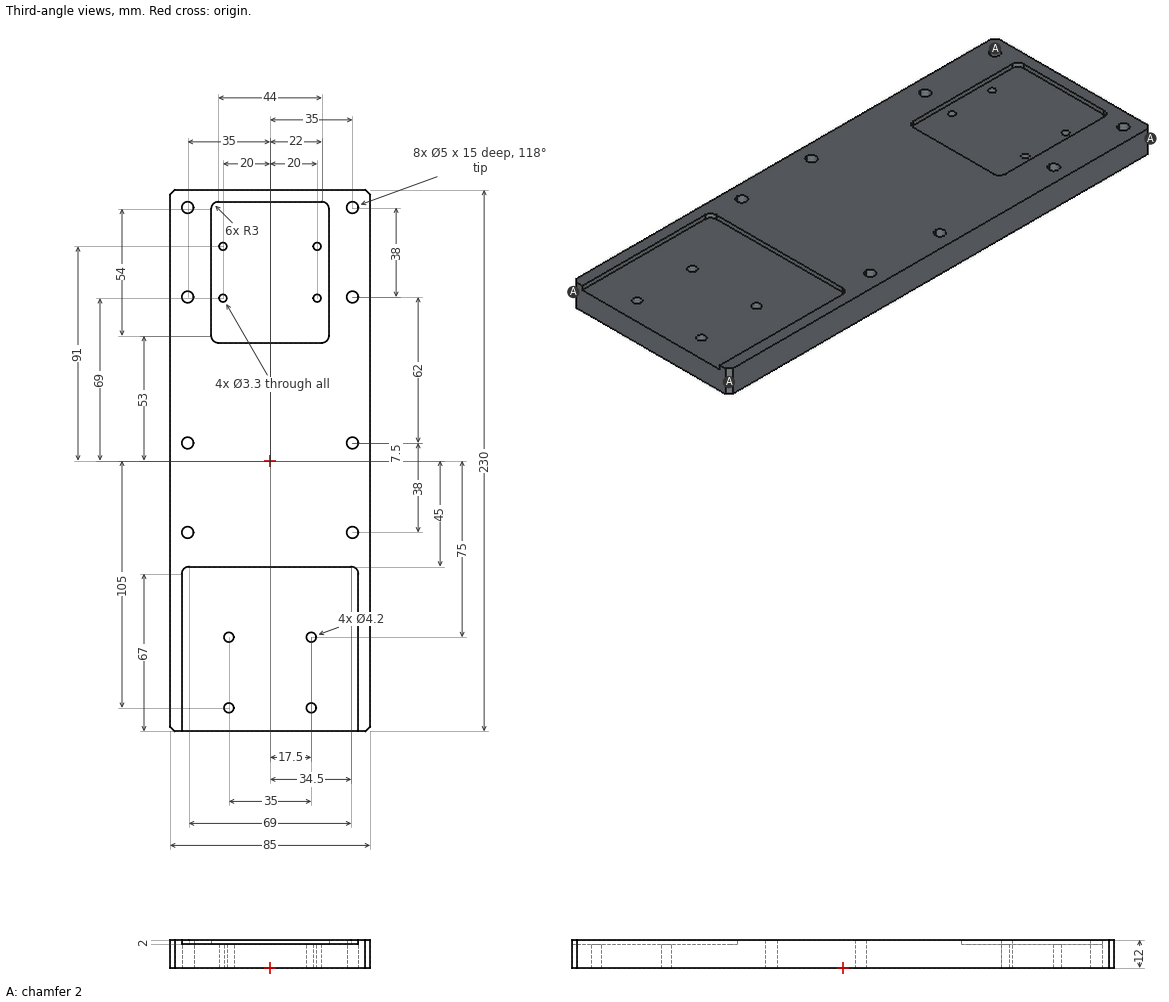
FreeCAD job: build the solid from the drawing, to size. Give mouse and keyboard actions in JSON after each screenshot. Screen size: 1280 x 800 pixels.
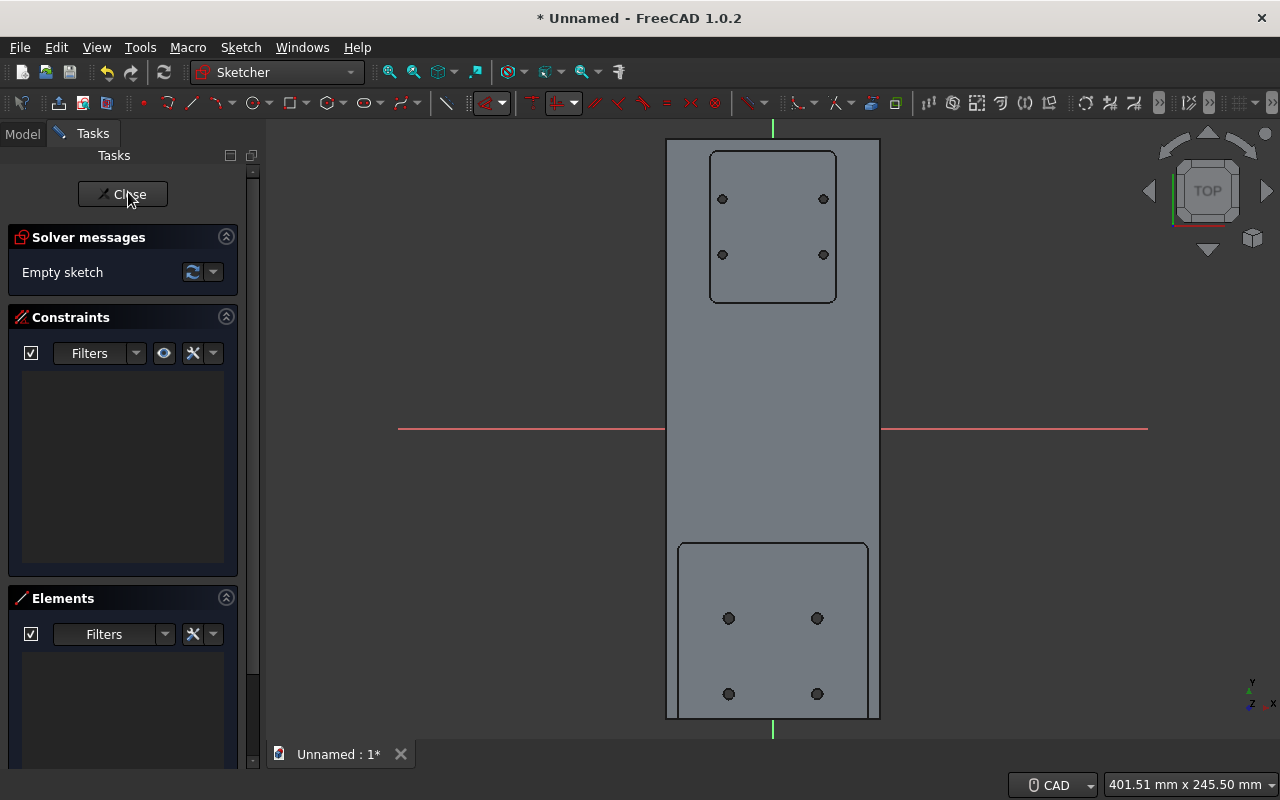
{"action": "key", "text": "q s"}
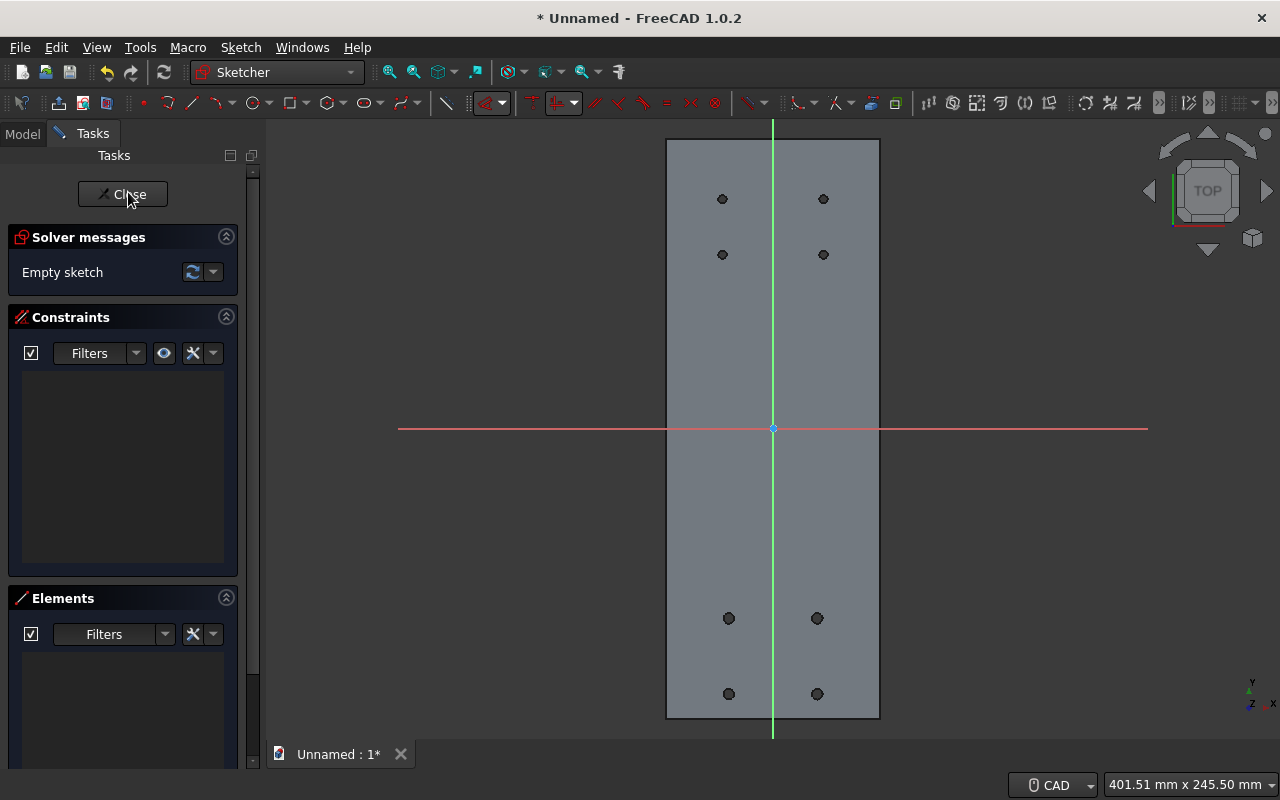
{"action": "scroll", "coordinate": [395, 711], "scroll_direction": "down", "scroll_amount": 1}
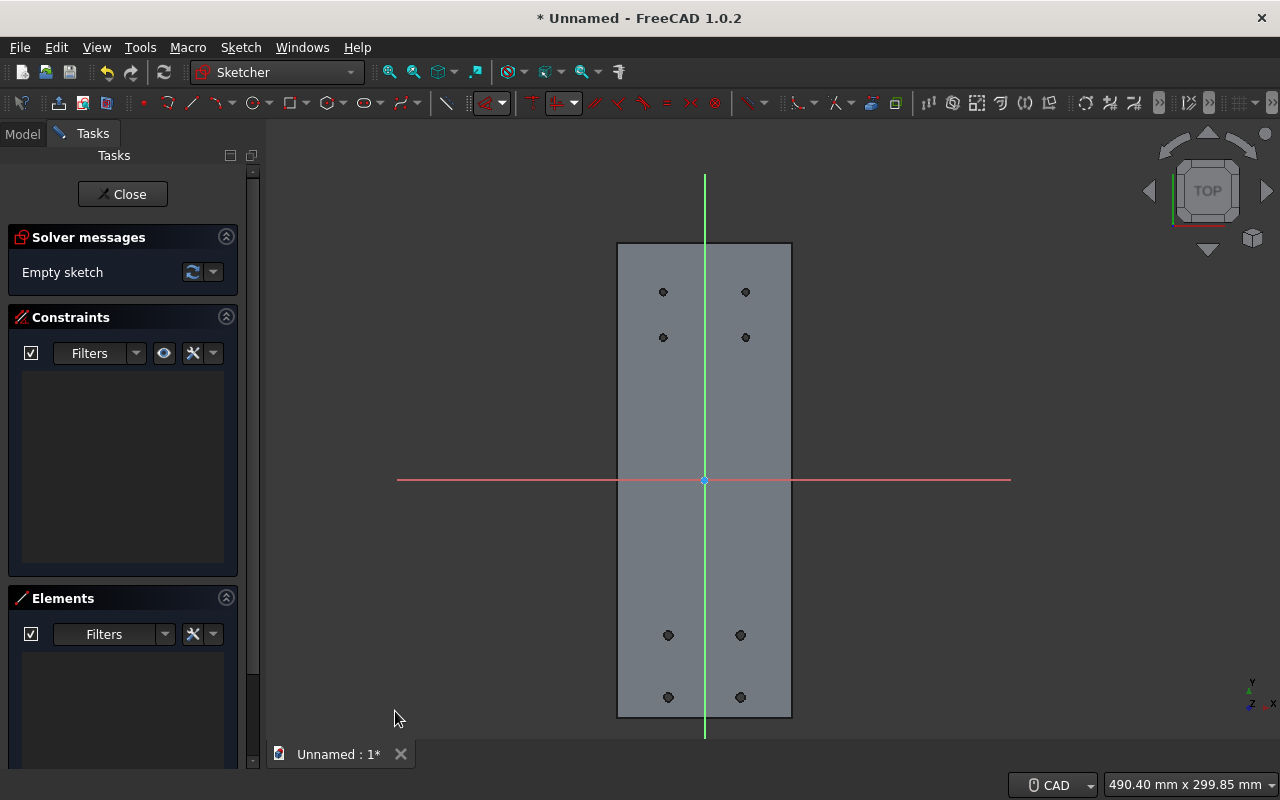
{"action": "key", "text": "g c"}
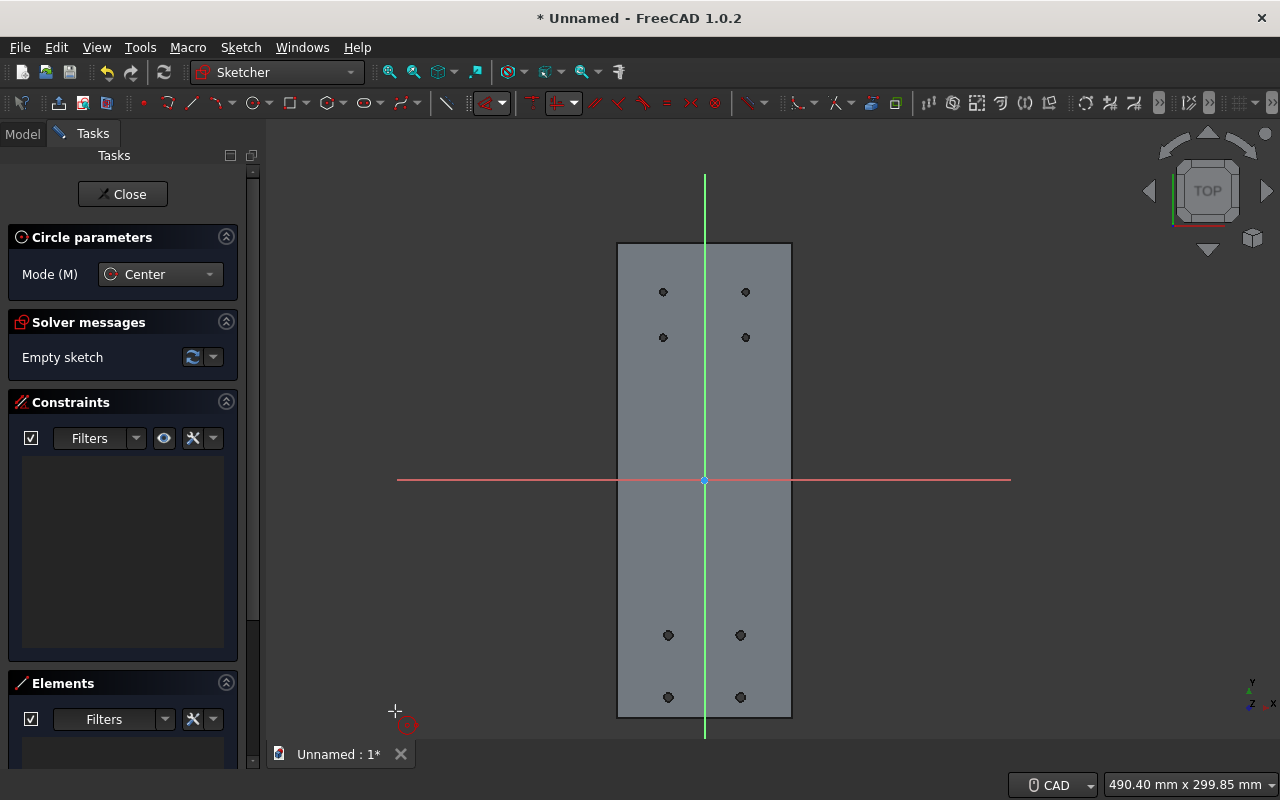
{"action": "scroll", "coordinate": [777, 258], "scroll_direction": "up", "scroll_amount": 8}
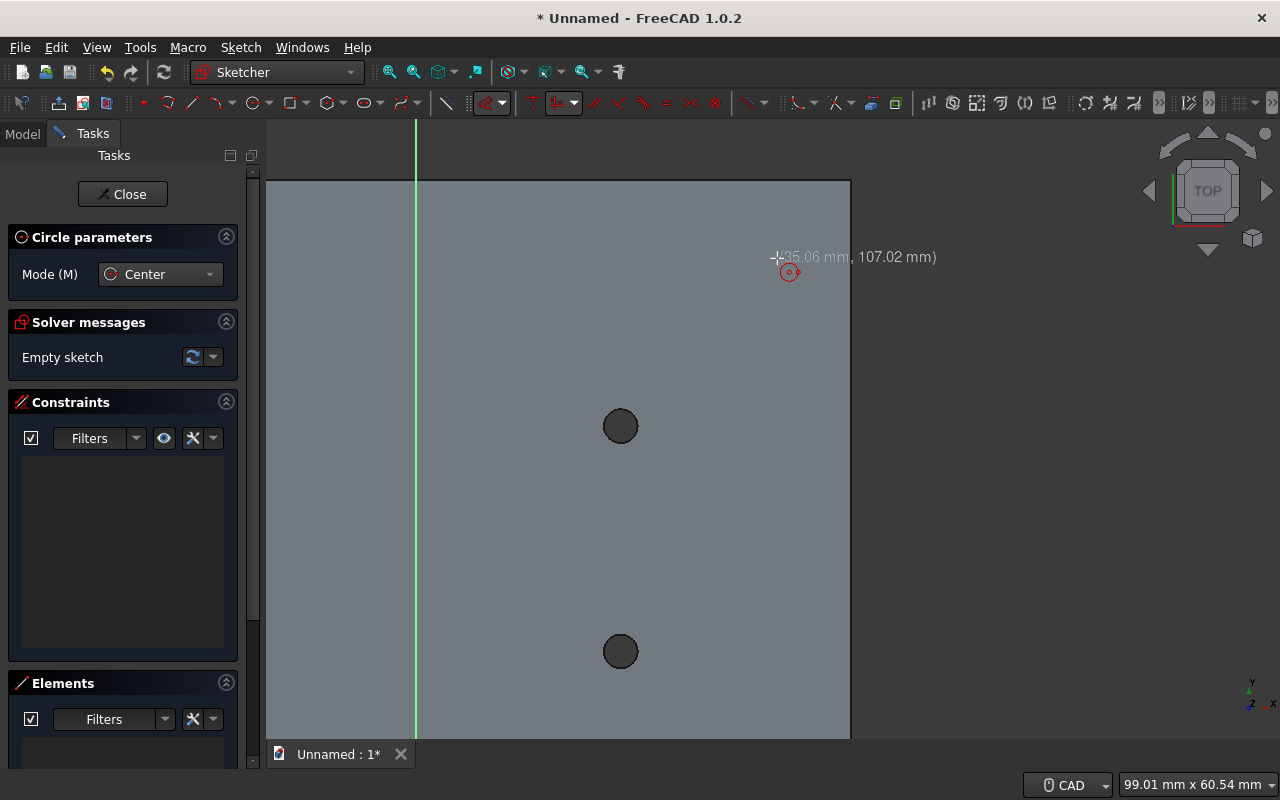
{"action": "scroll", "coordinate": [799, 254], "scroll_direction": "down", "scroll_amount": 7}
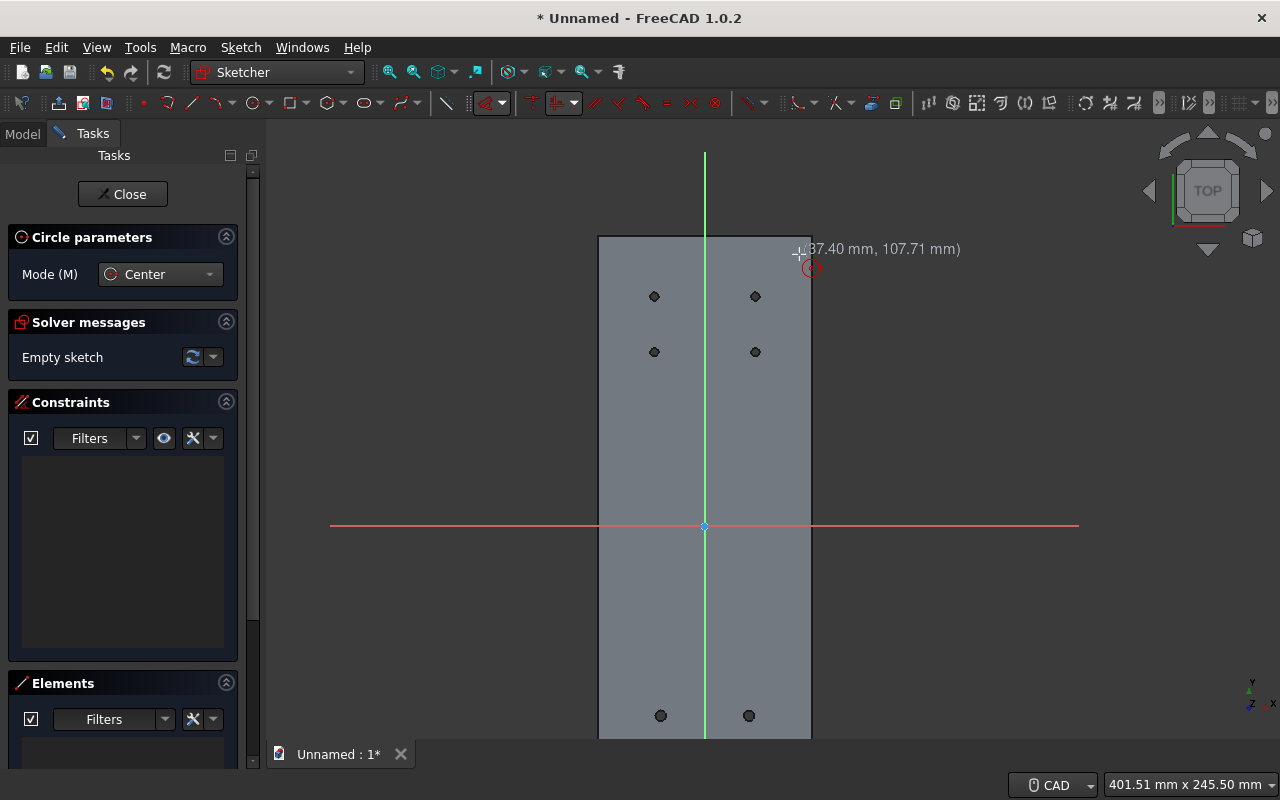
{"action": "left_click", "coordinate": [793, 255]}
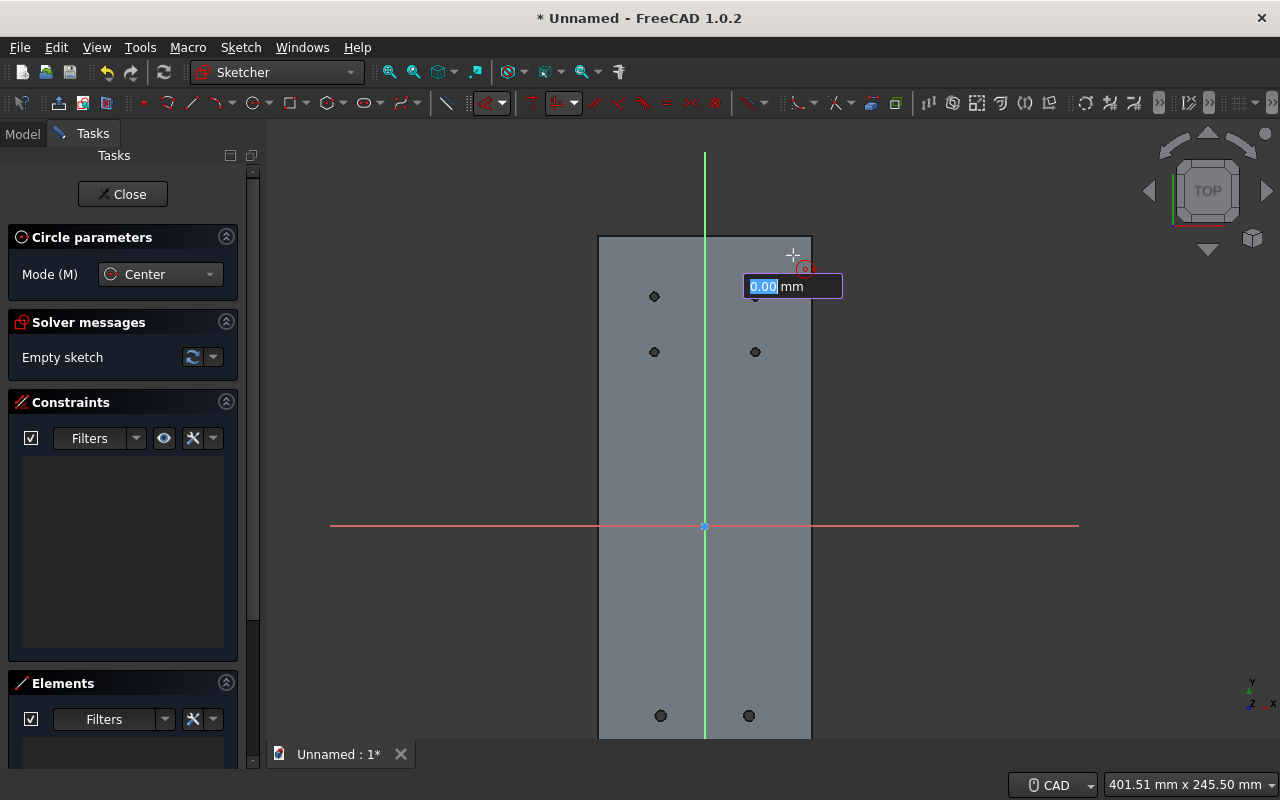
{"action": "scroll", "coordinate": [798, 250], "scroll_direction": "up", "scroll_amount": 5}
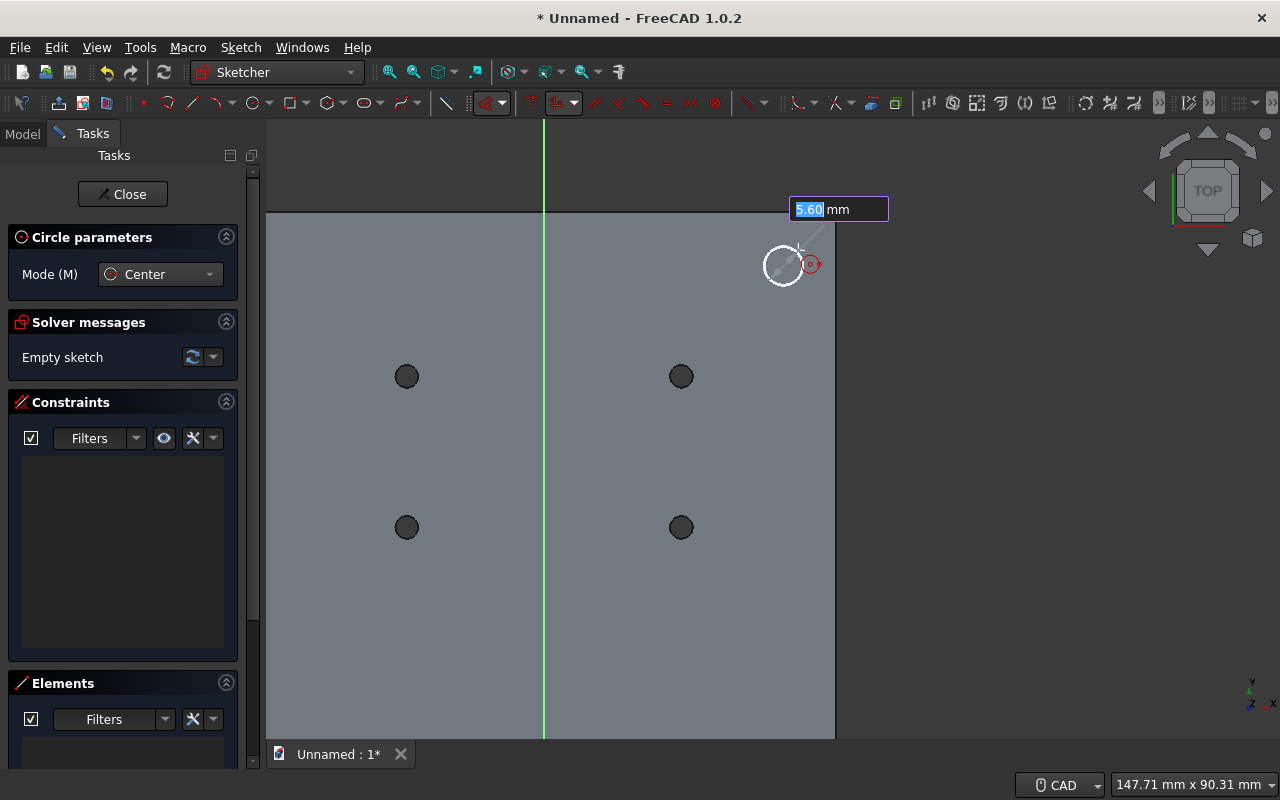
{"action": "left_click", "coordinate": [797, 251]}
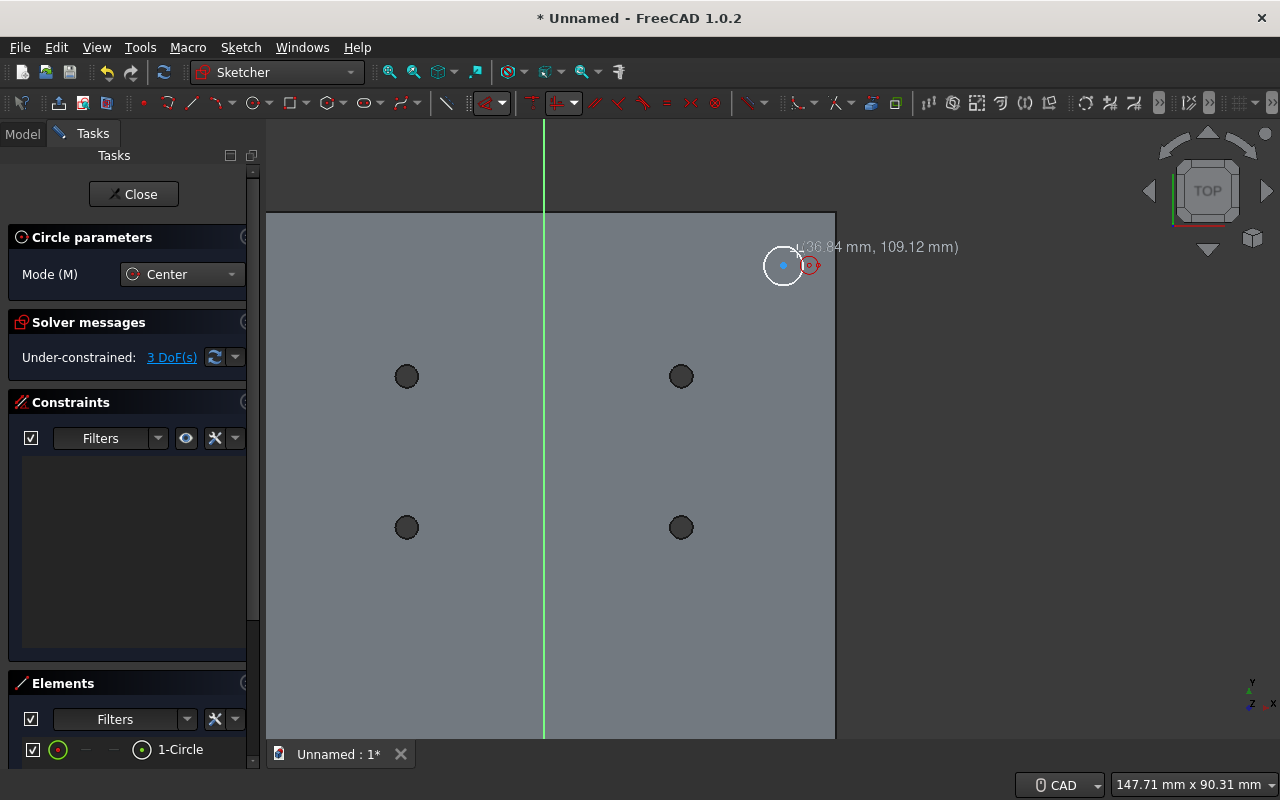
{"action": "scroll", "coordinate": [784, 524], "scroll_direction": "up", "scroll_amount": 2}